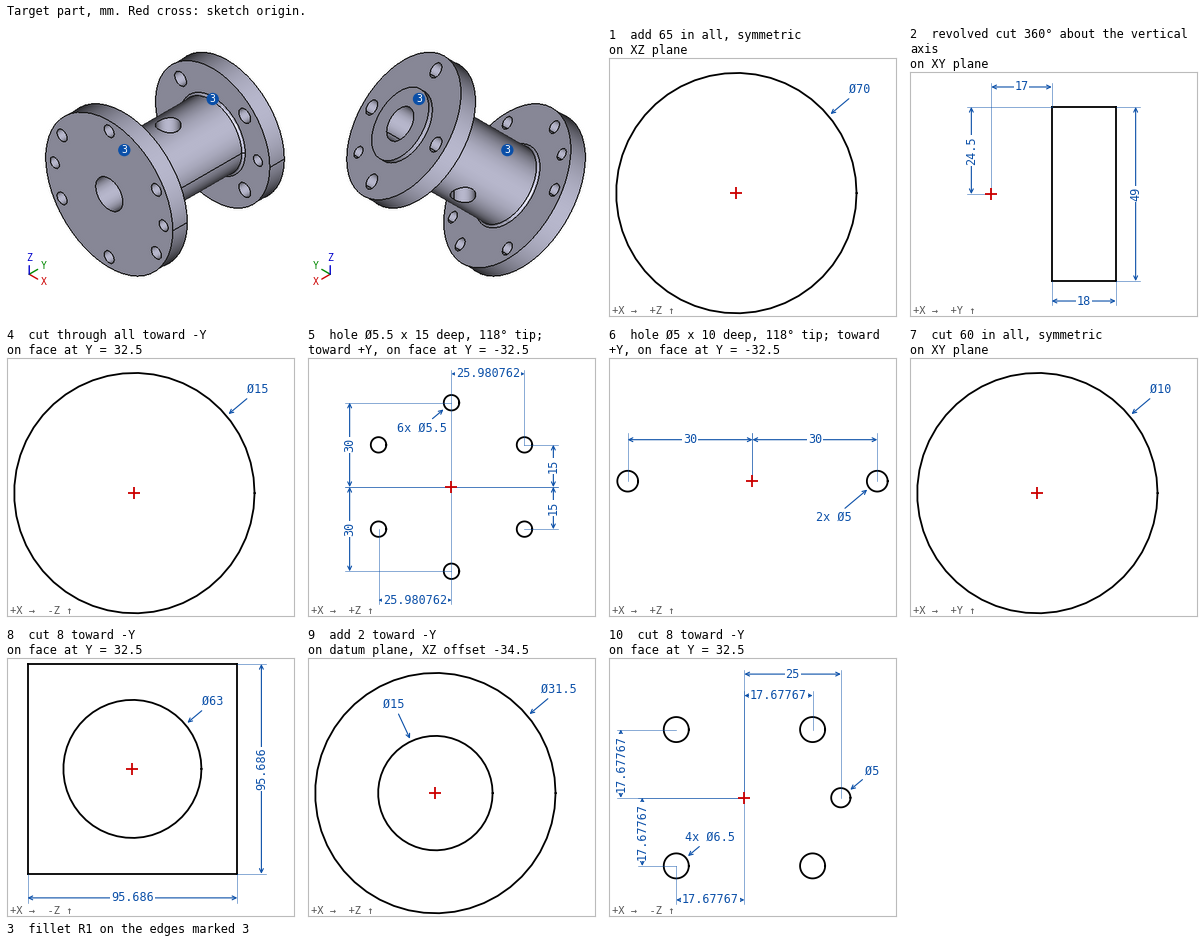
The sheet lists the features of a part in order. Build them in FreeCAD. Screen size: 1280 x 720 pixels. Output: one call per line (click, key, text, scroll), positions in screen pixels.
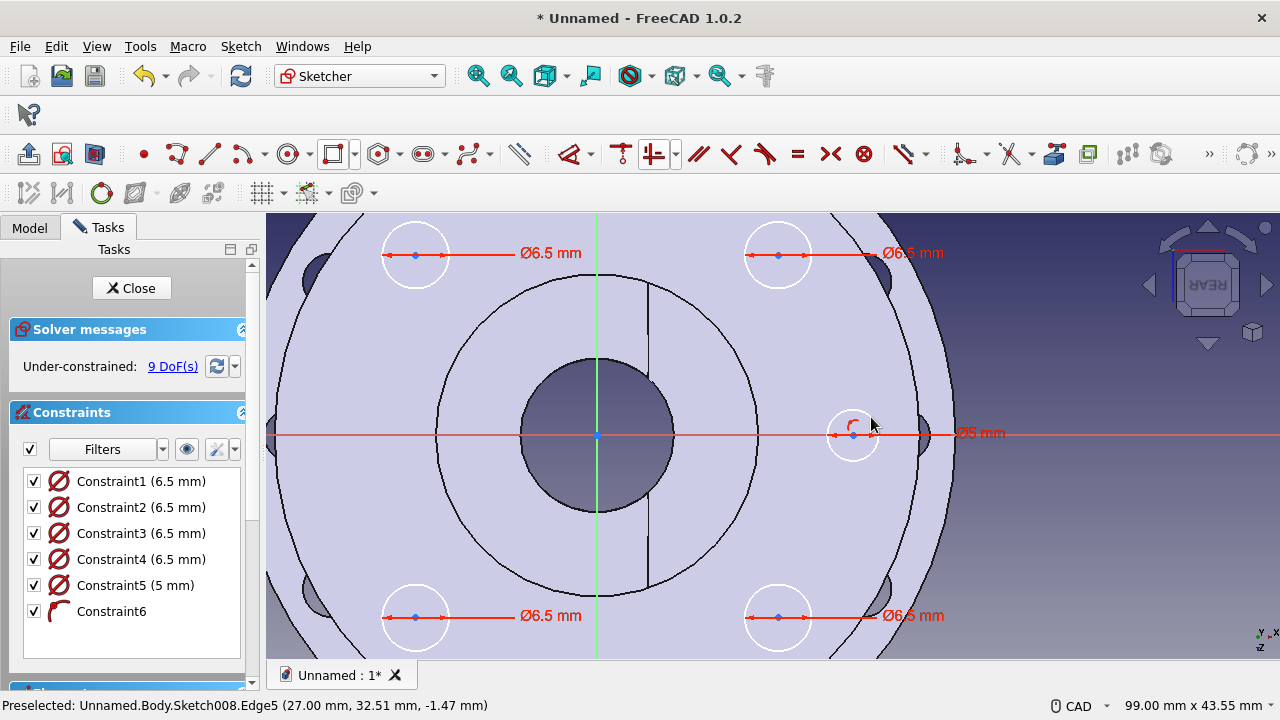
click(416, 618)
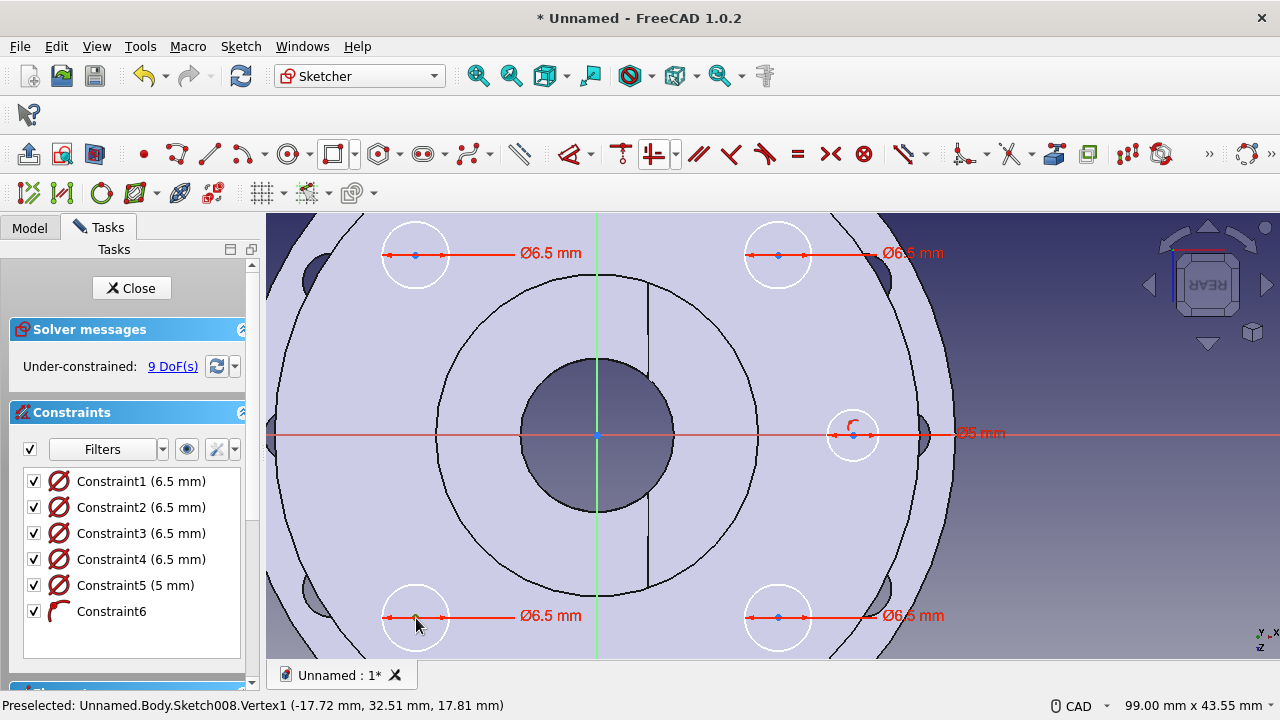
click(416, 255)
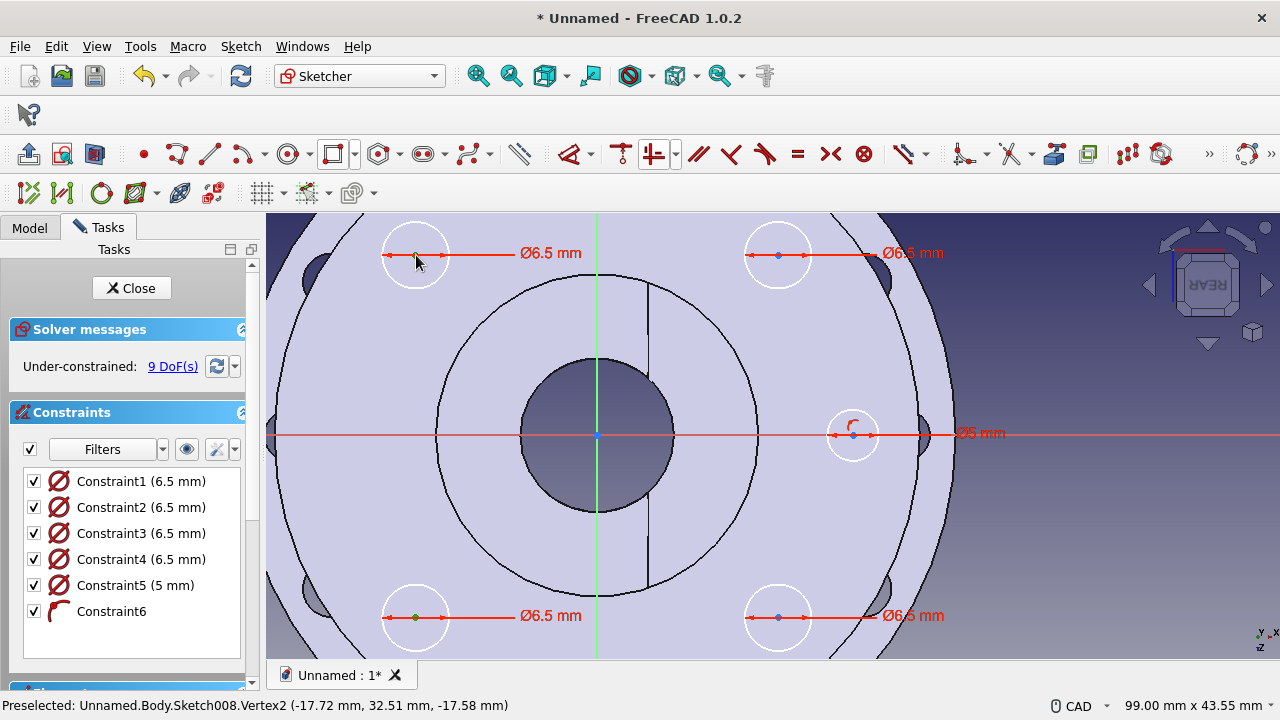
click(676, 154)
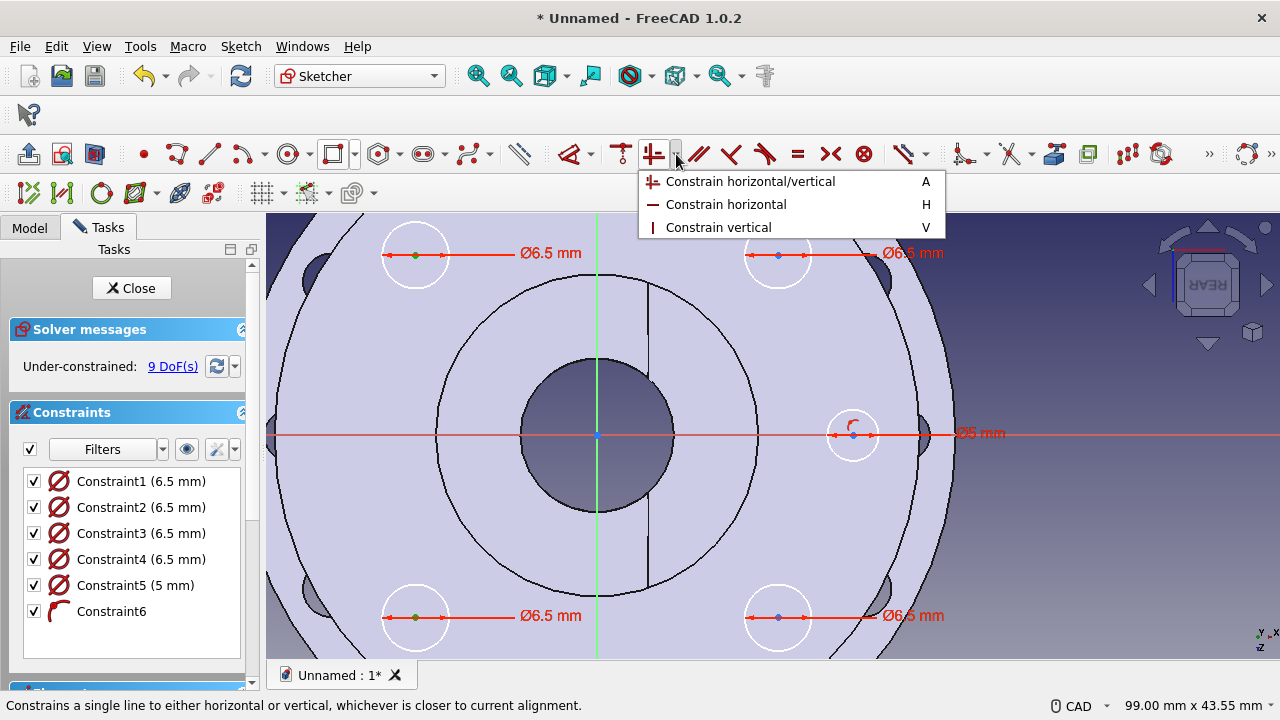
click(792, 228)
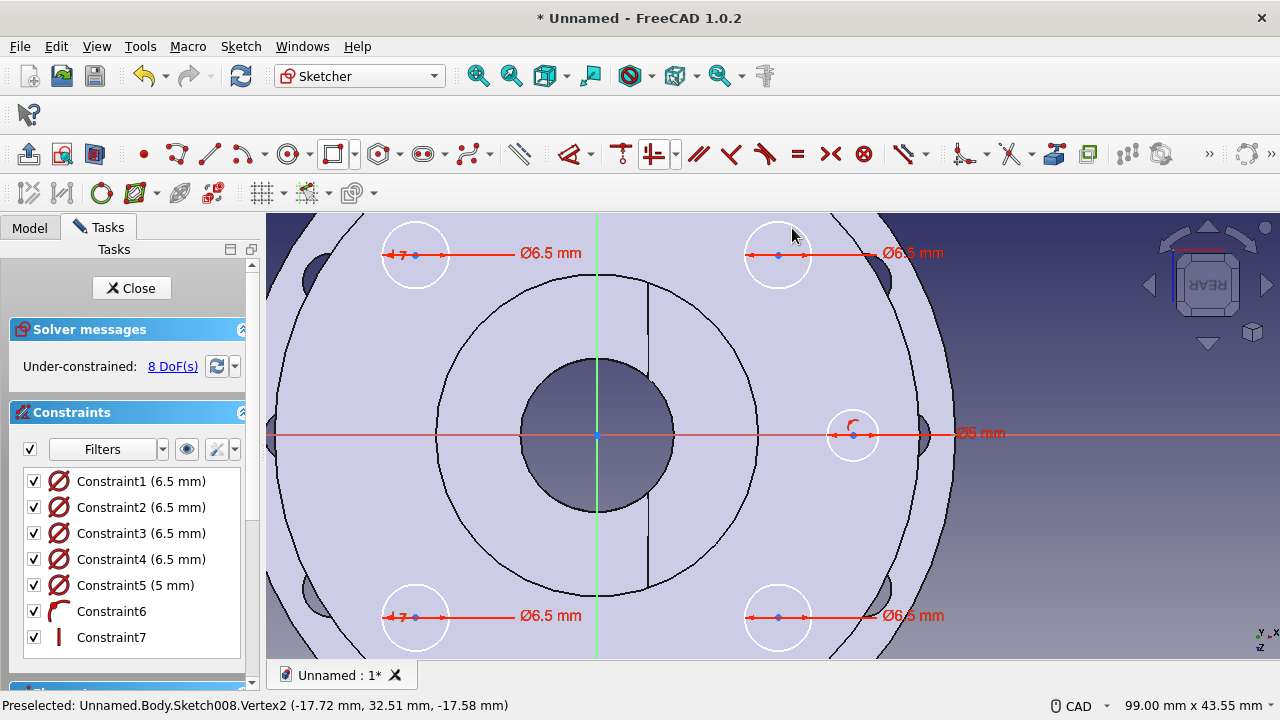
click(416, 255)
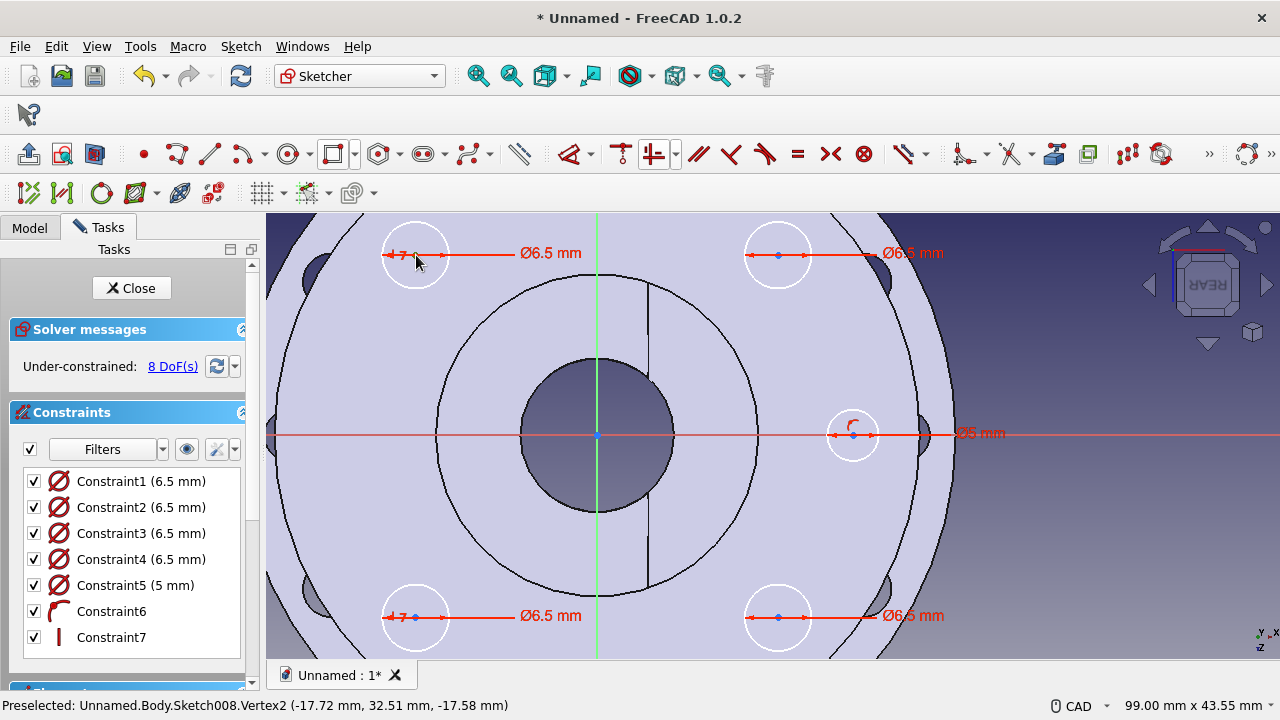
click(778, 255)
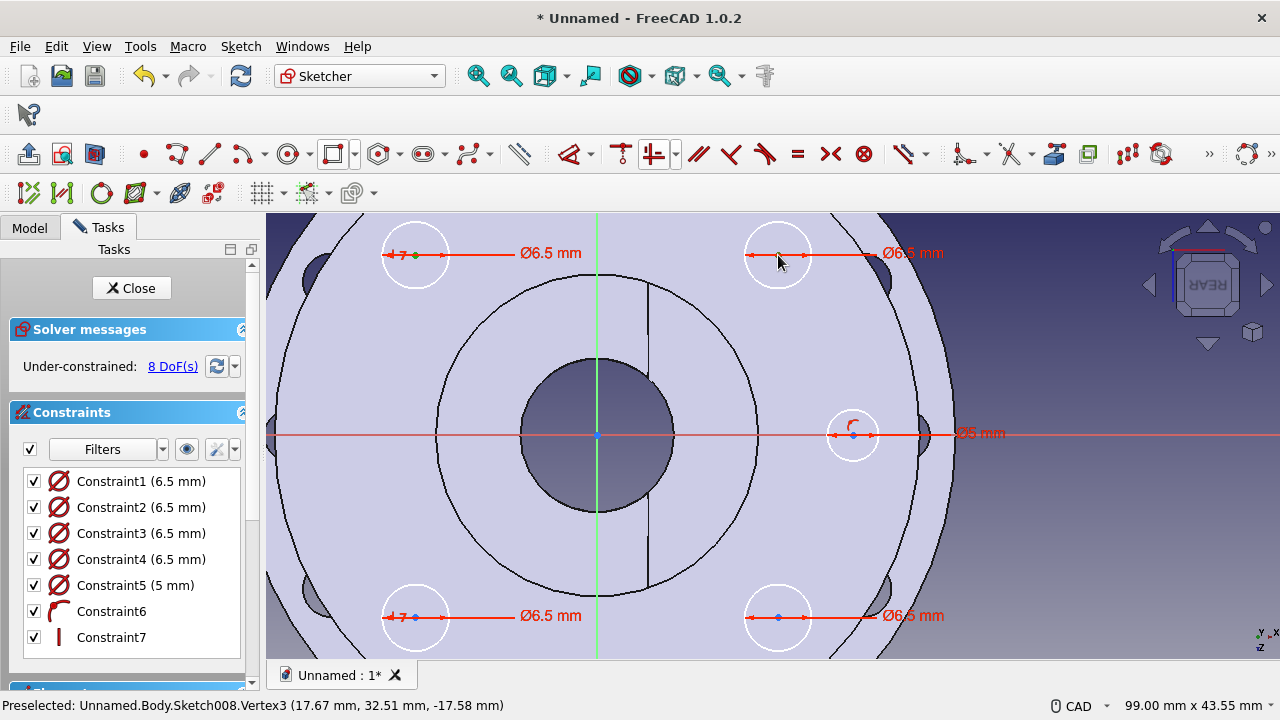
click(676, 154)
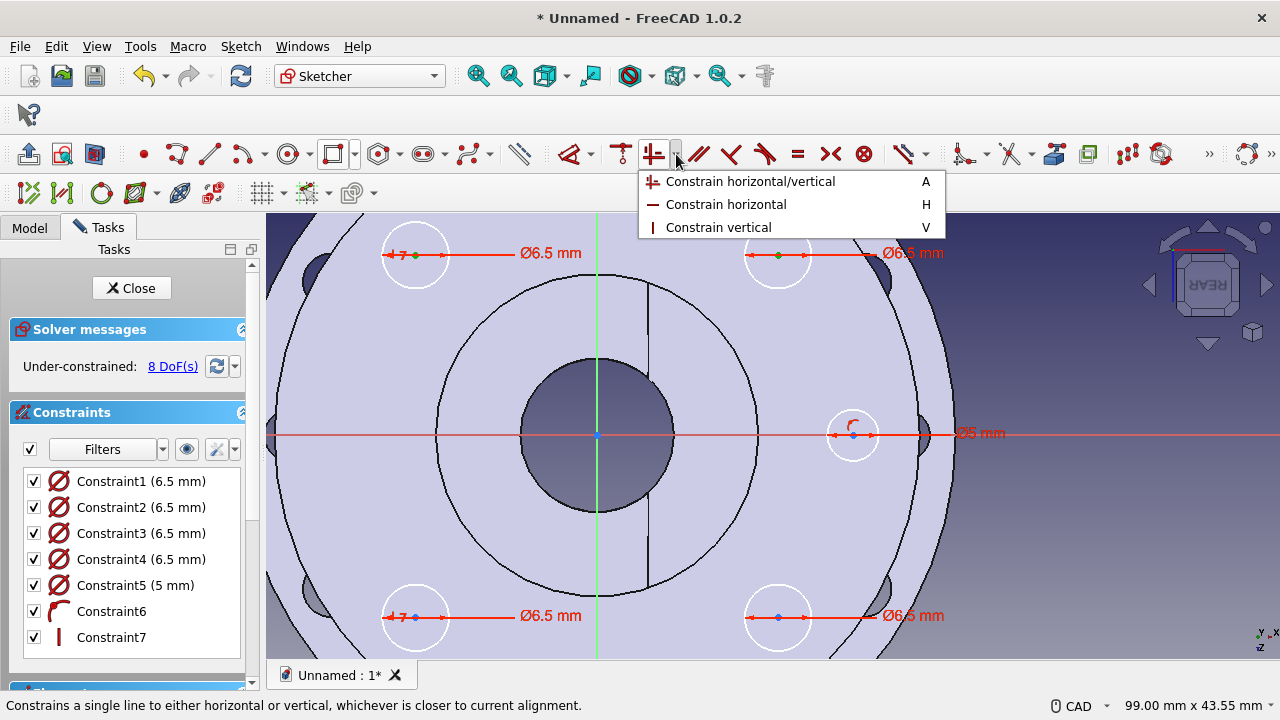
click(792, 204)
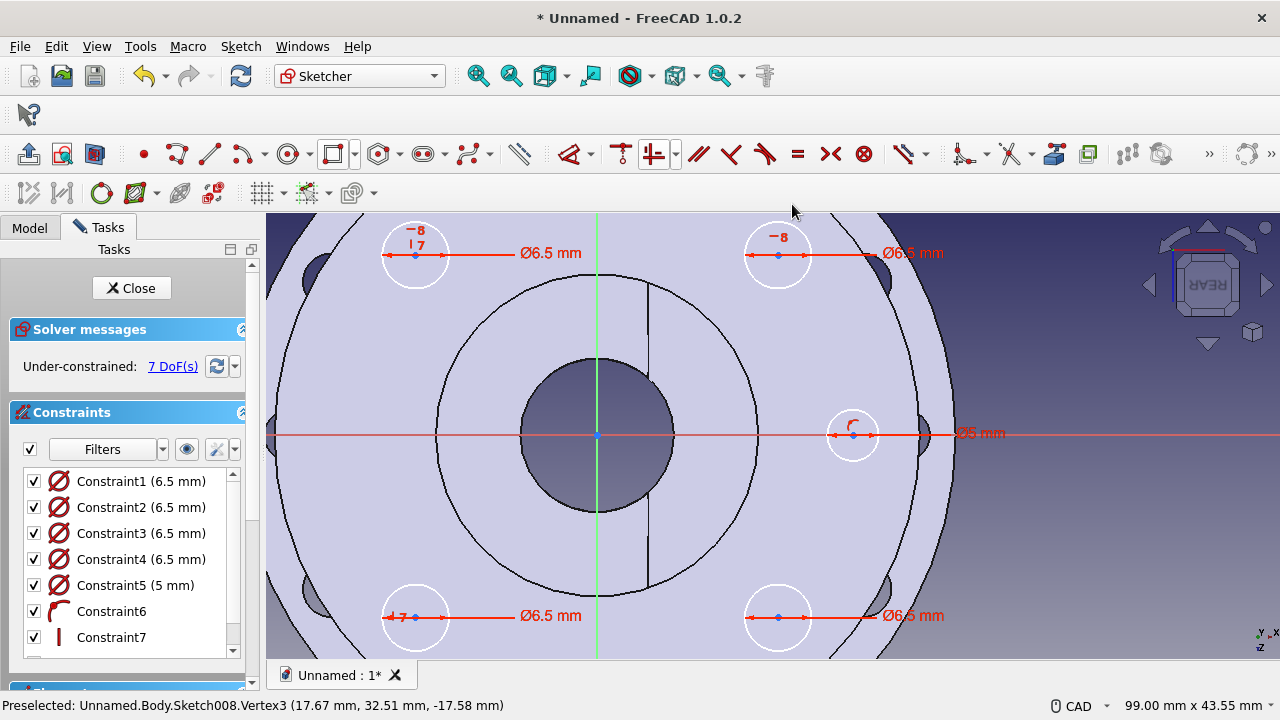
click(778, 255)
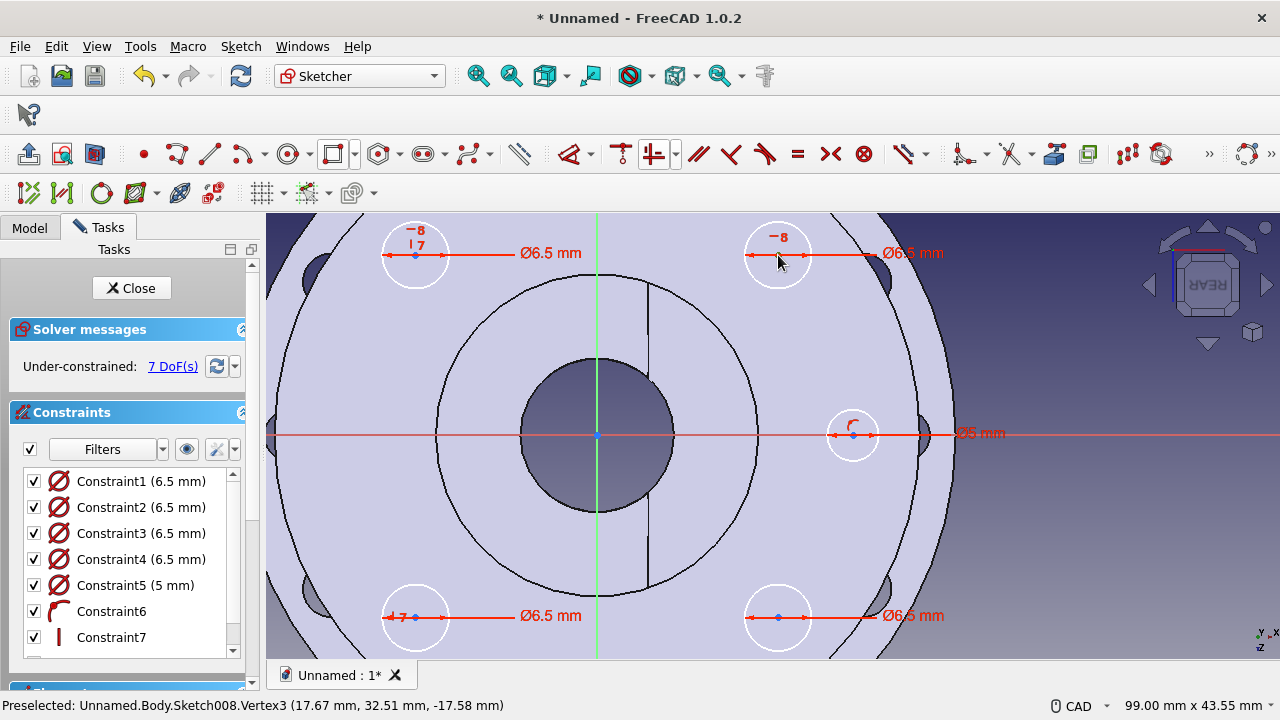
click(778, 618)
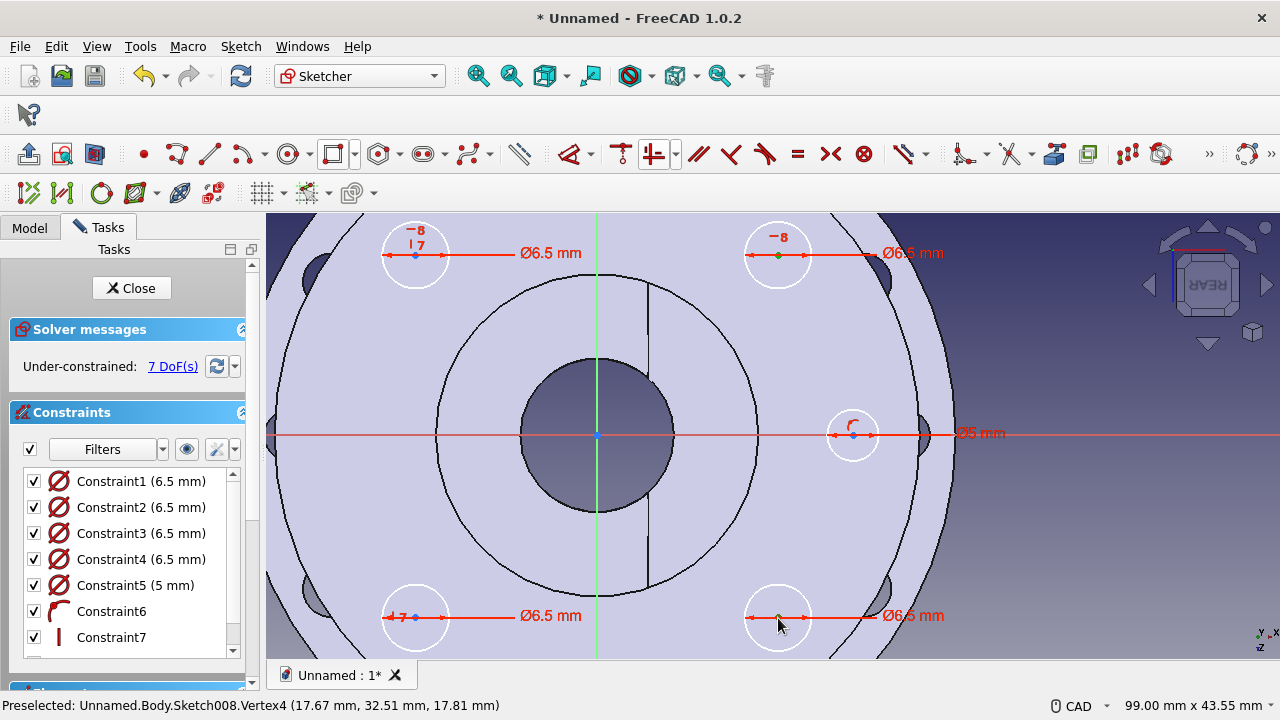
click(676, 154)